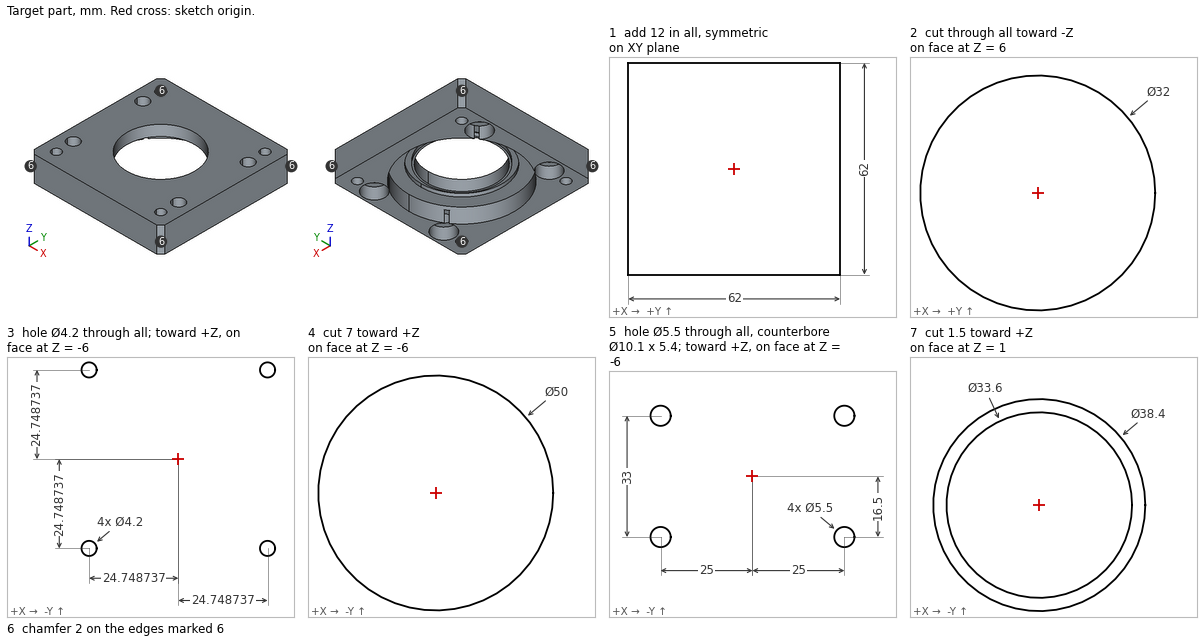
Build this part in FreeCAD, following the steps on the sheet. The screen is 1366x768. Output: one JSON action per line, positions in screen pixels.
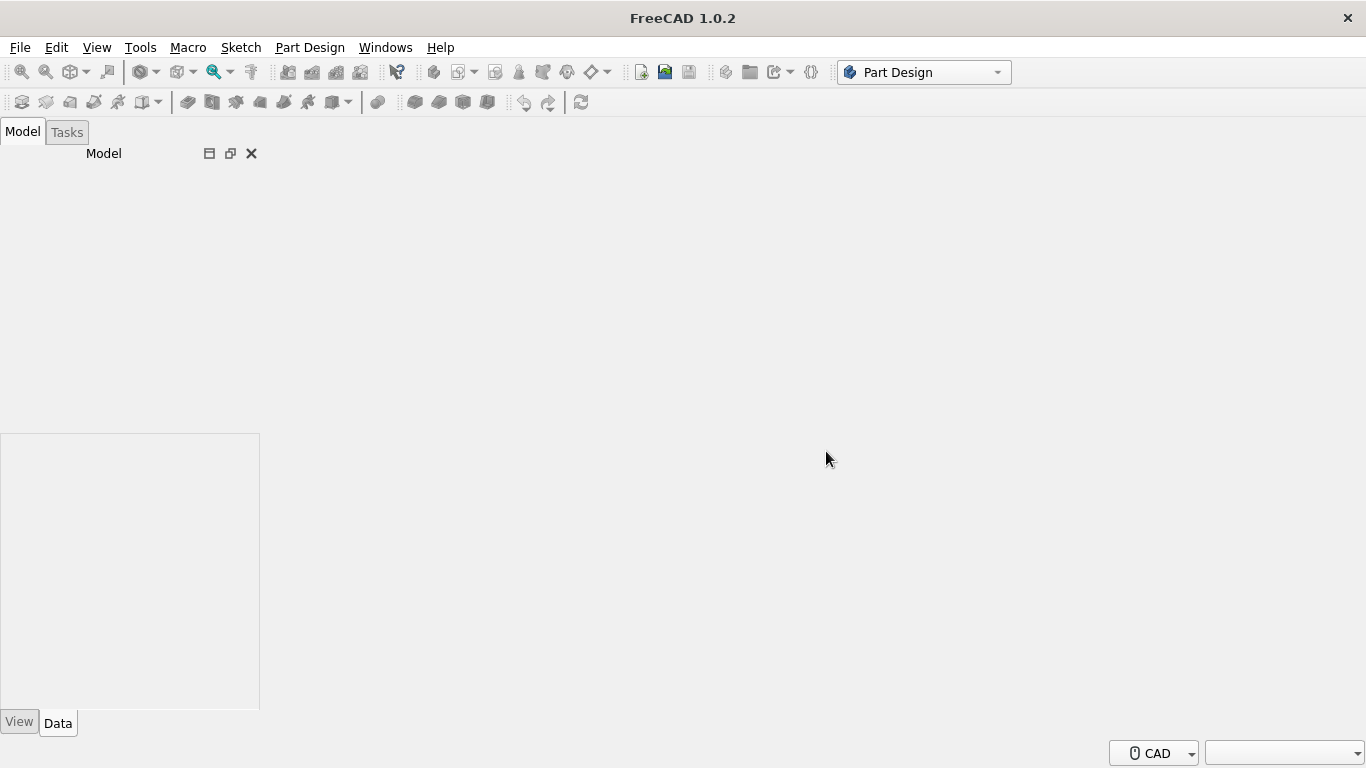
{"action": "left_click", "coordinate": [642, 72]}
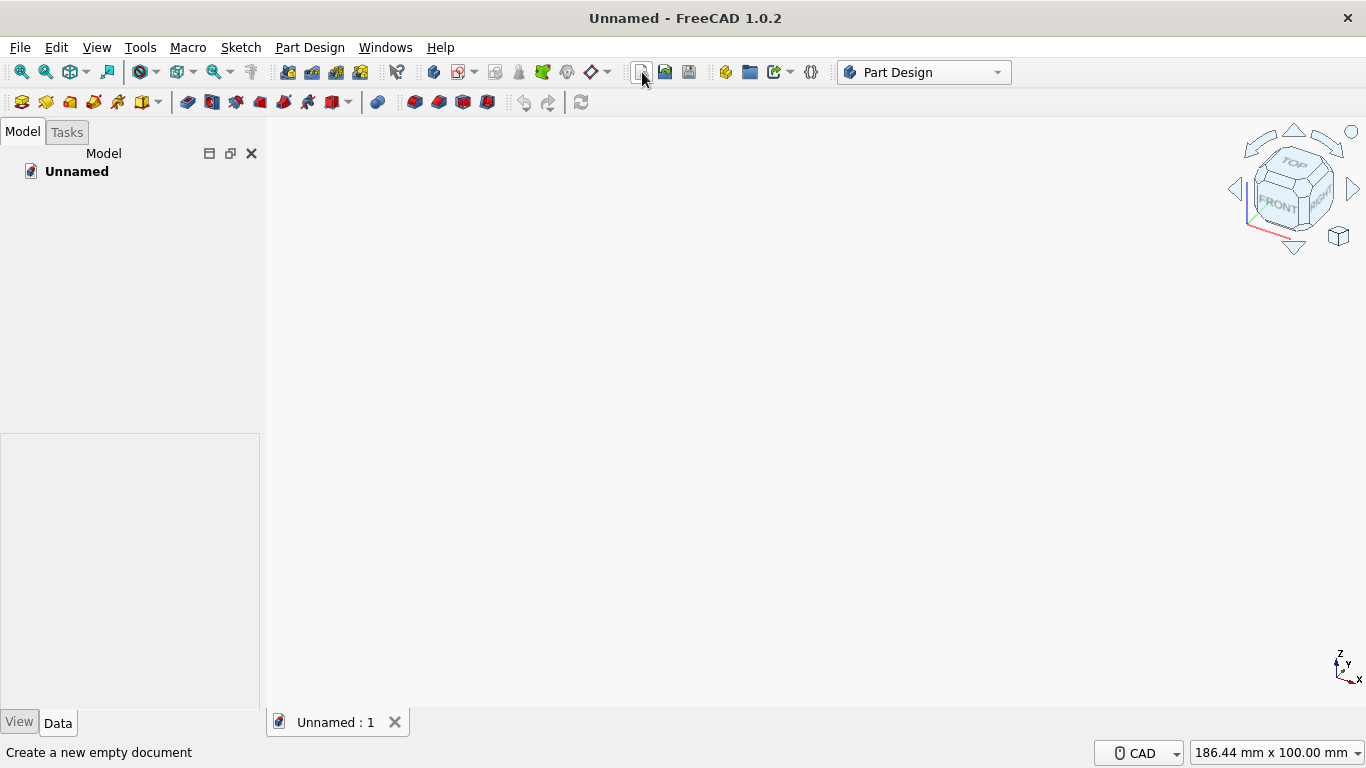
{"action": "left_click", "coordinate": [458, 72]}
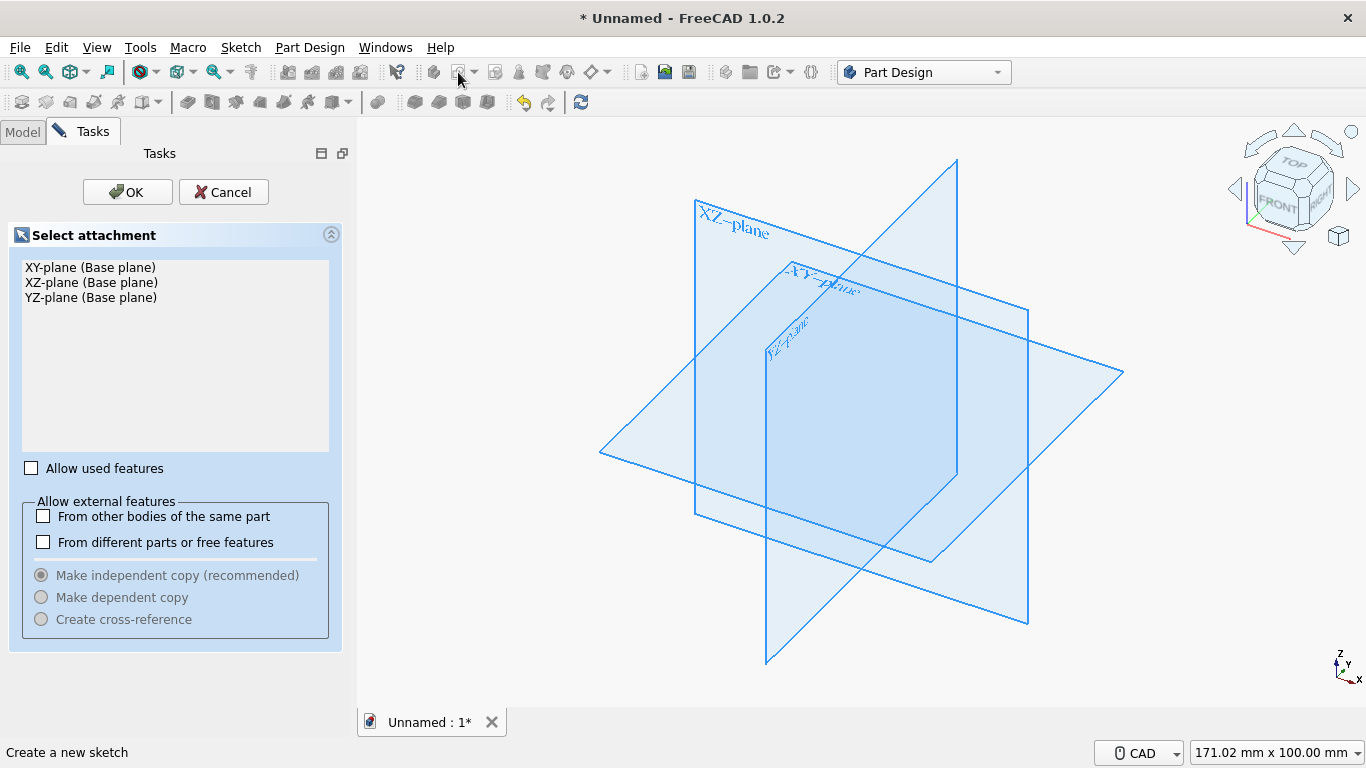
{"action": "left_click", "coordinate": [82, 268]}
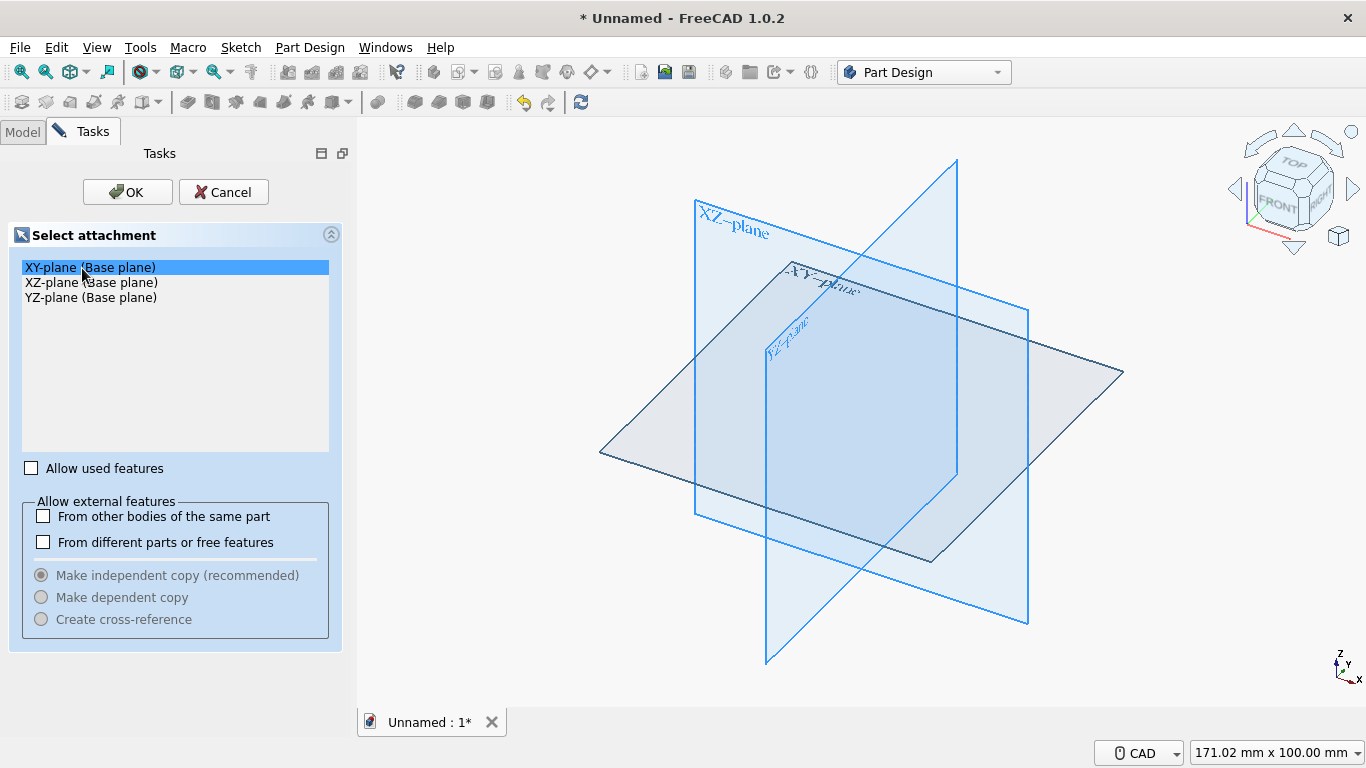
{"action": "left_click", "coordinate": [128, 192]}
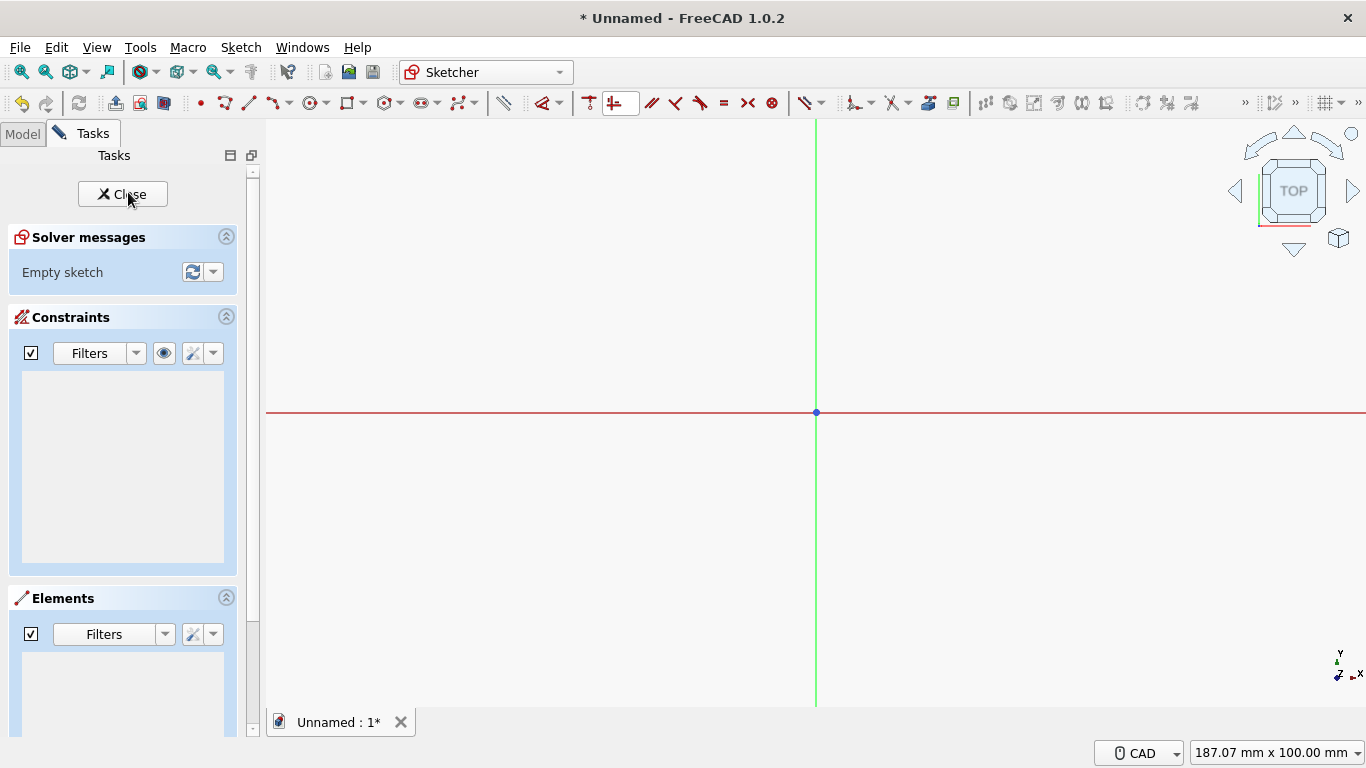
{"action": "left_click", "coordinate": [366, 104]}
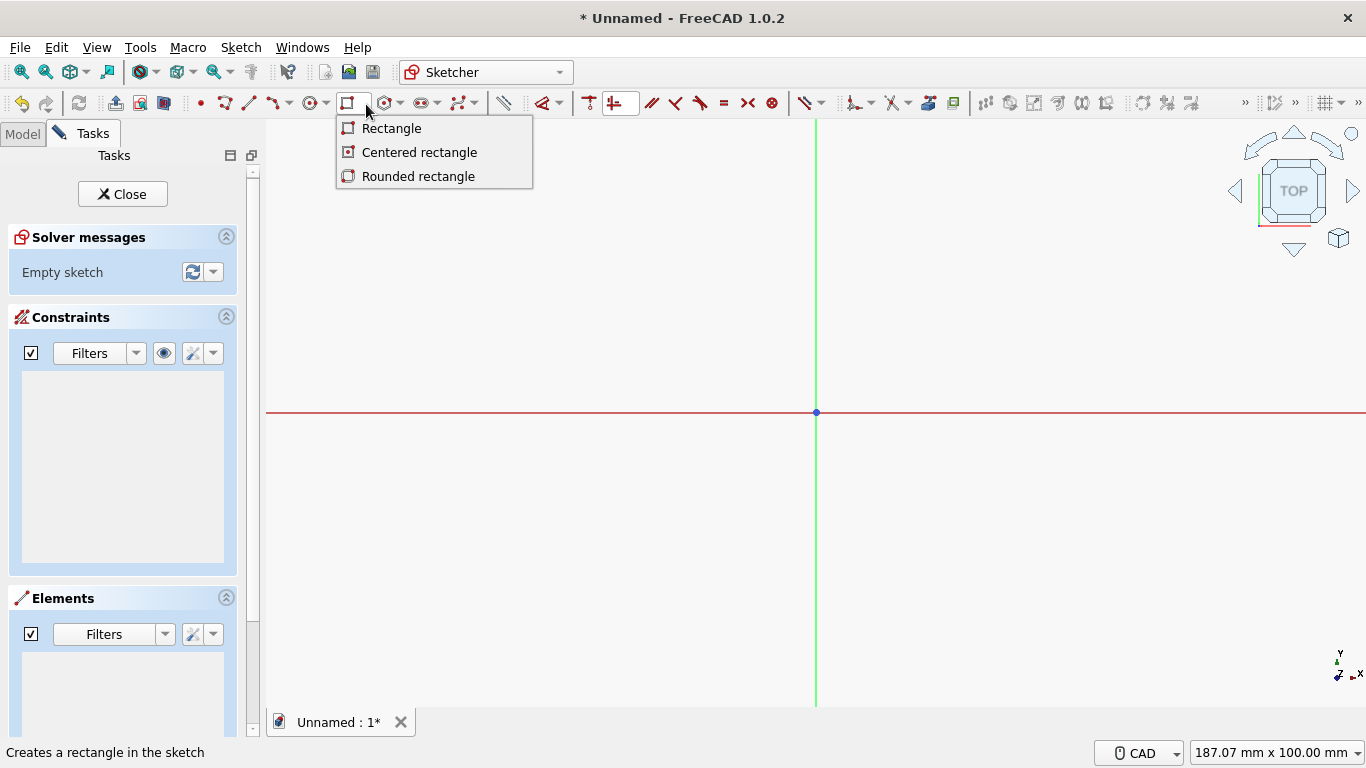
{"action": "left_click", "coordinate": [434, 152]}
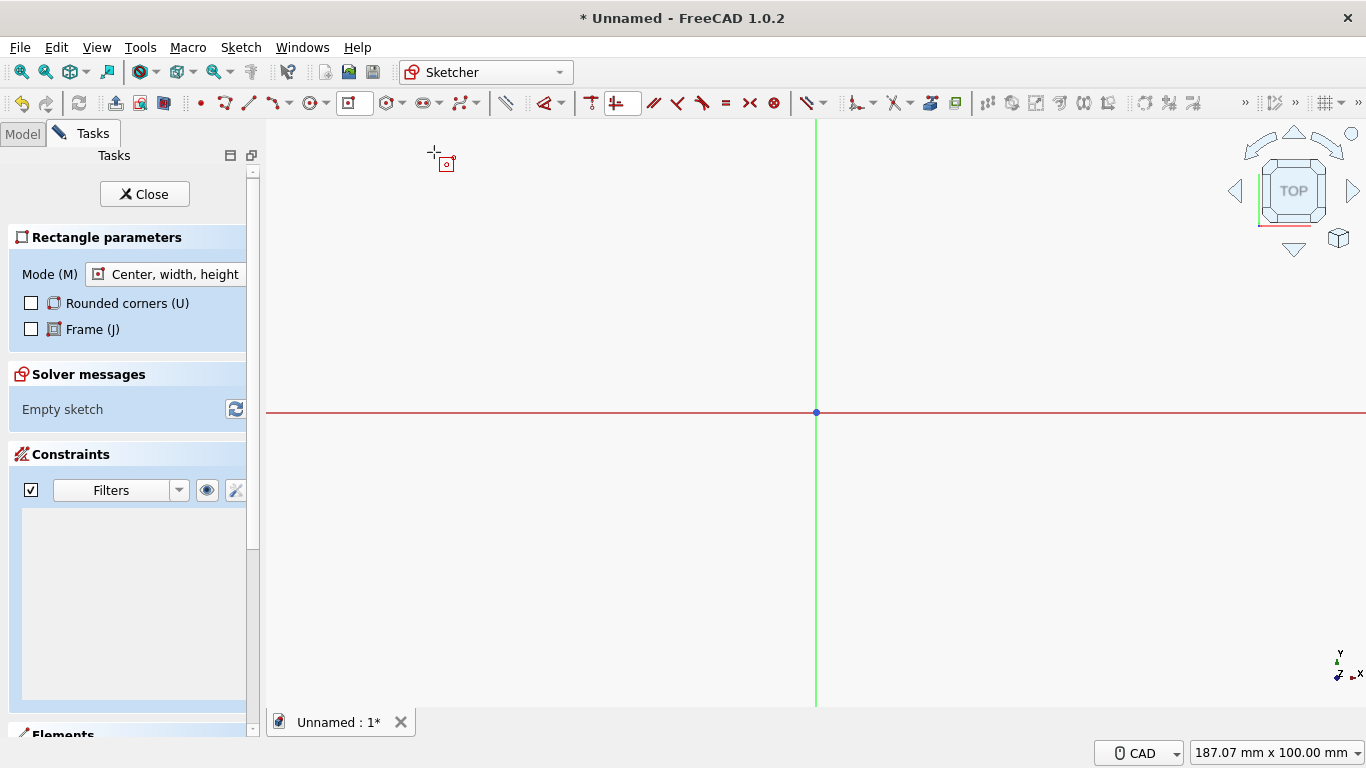
{"action": "left_click", "coordinate": [816, 413]}
{"action": "mouse_move", "coordinate": [998, 231]}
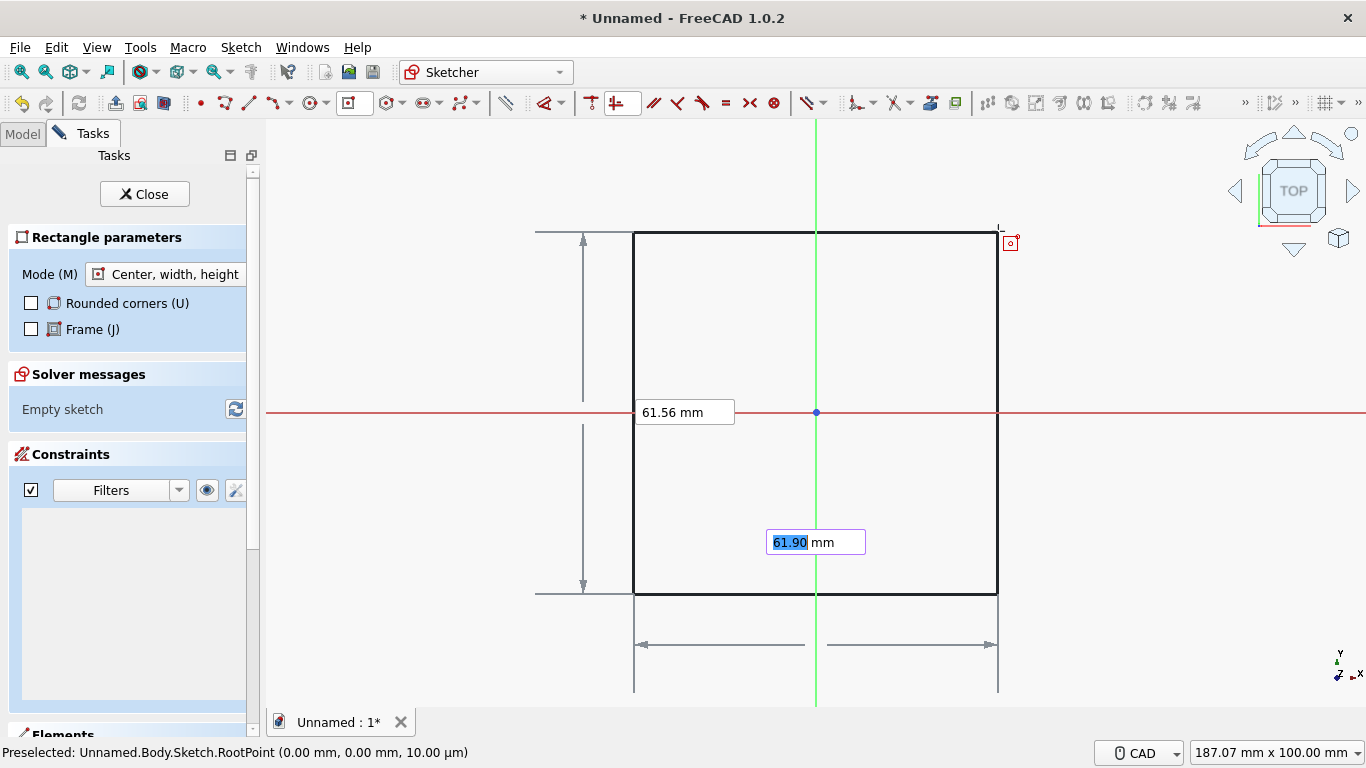
{"action": "type", "text": "62"}
{"action": "key", "text": "Tab"}
{"action": "type", "text": "62"}
{"action": "key", "text": "Return"}
{"action": "key", "text": "Escape"}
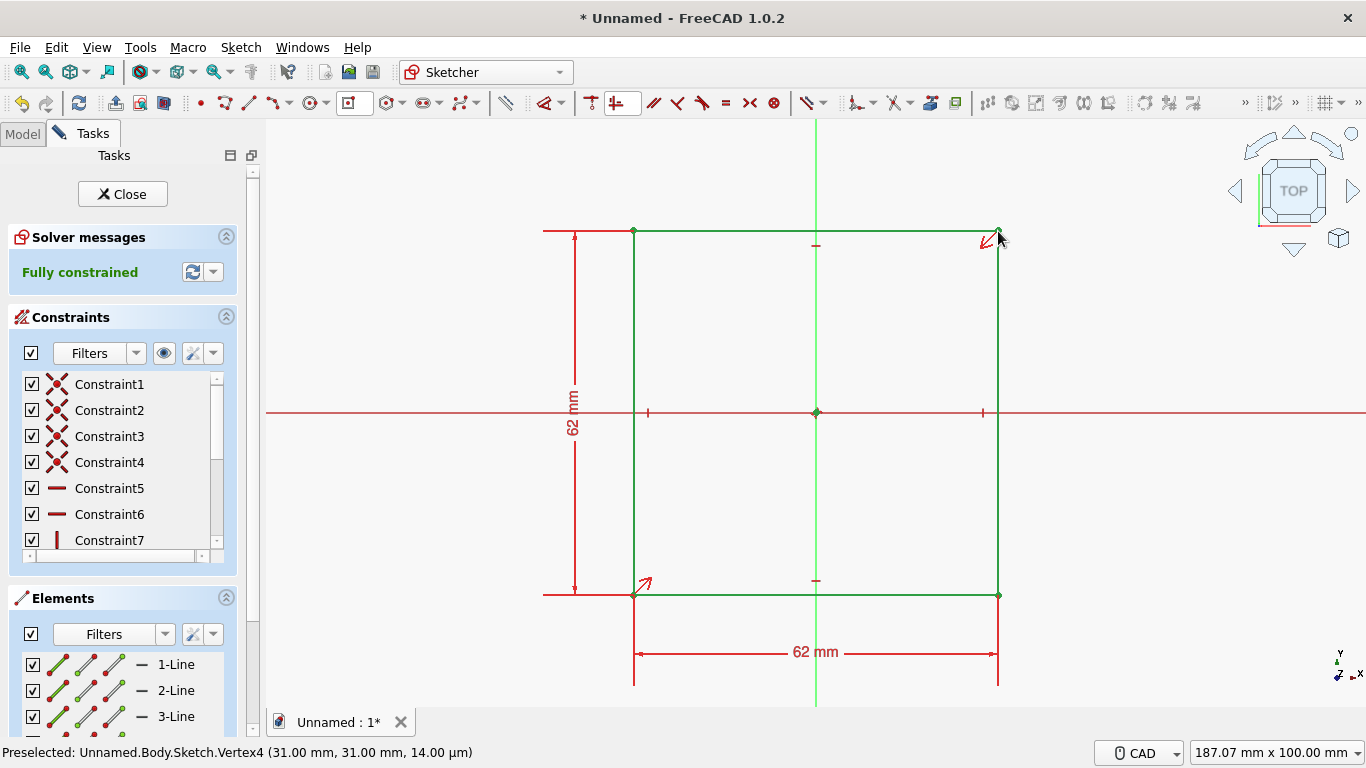
{"action": "left_click", "coordinate": [123, 194]}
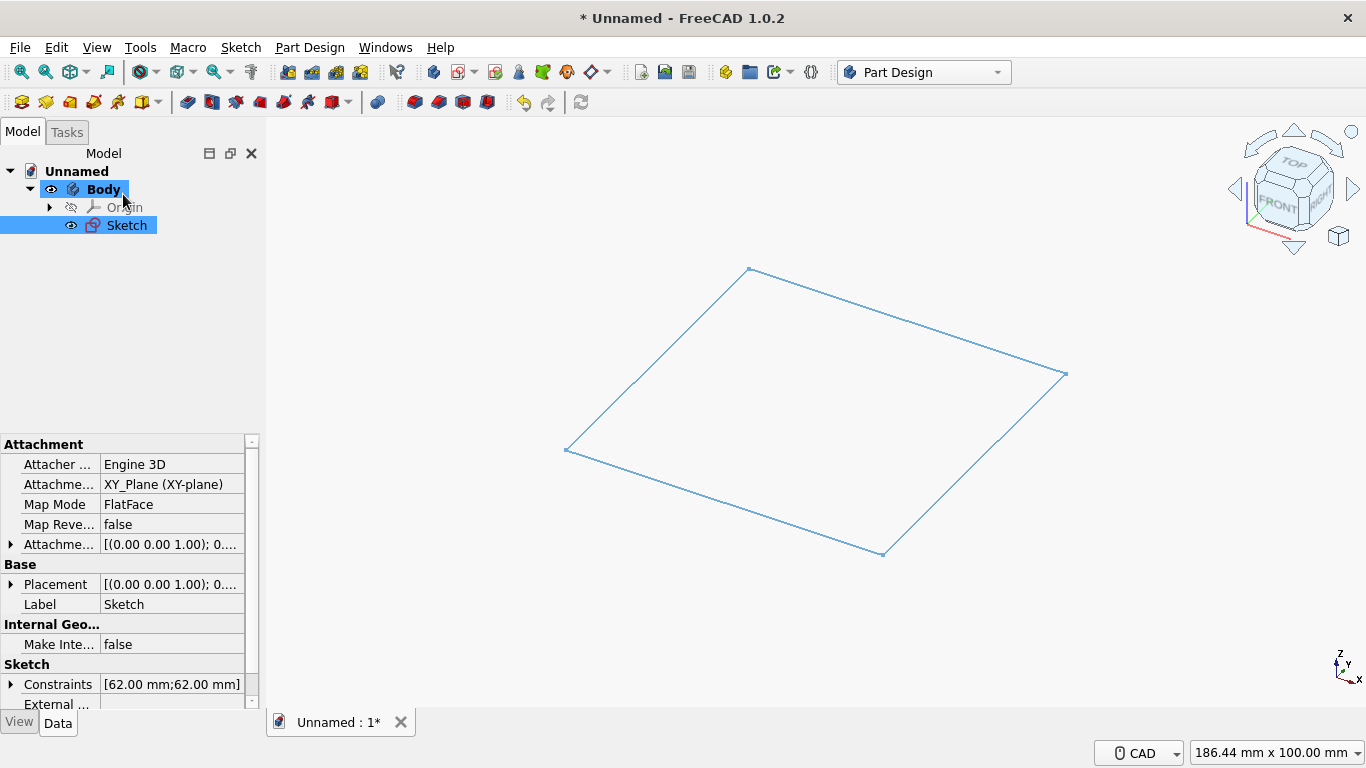
{"action": "left_click", "coordinate": [22, 102]}